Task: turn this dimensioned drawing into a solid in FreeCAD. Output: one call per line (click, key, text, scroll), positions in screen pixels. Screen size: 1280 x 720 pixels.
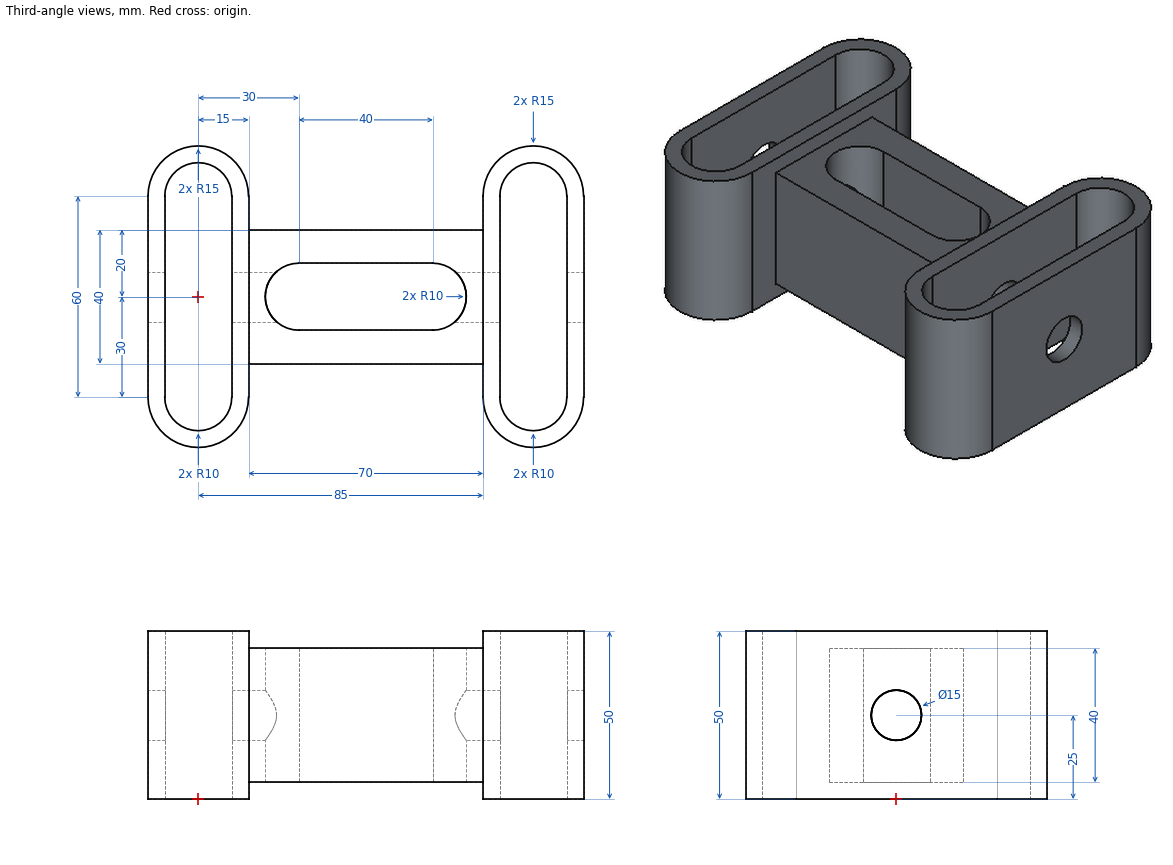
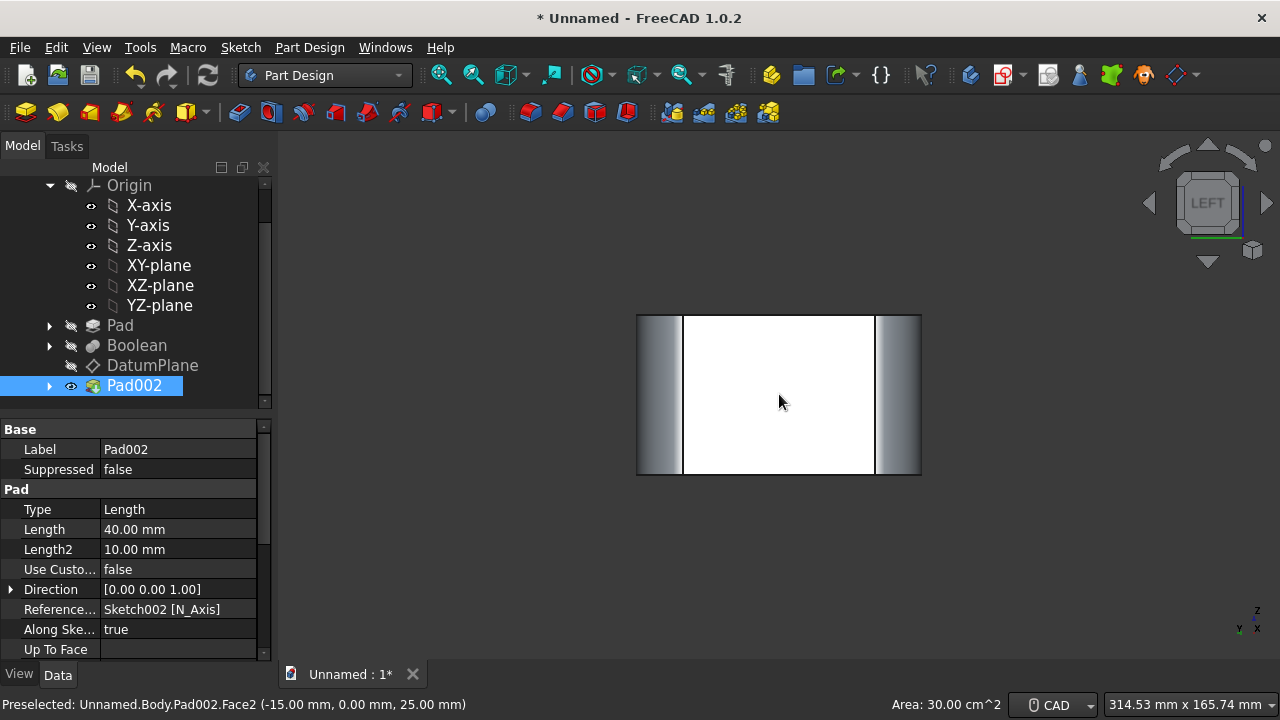
click(1004, 76)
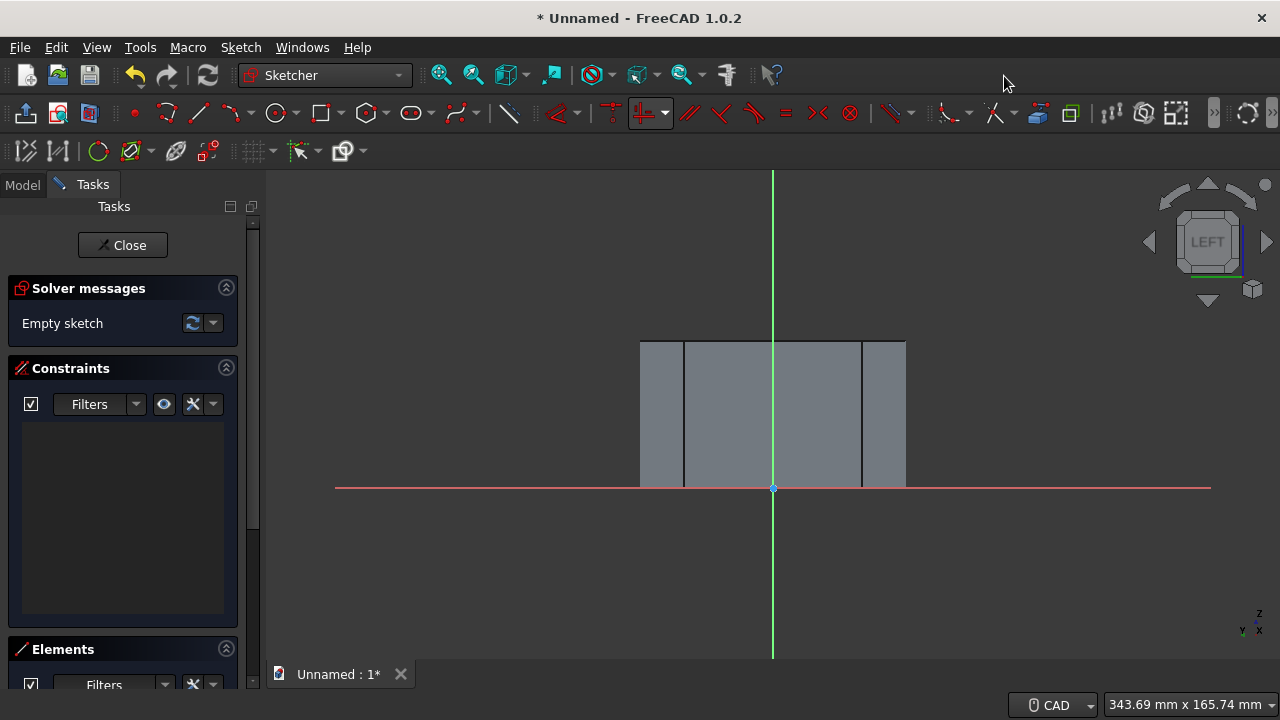
scroll(803, 451, up, 6)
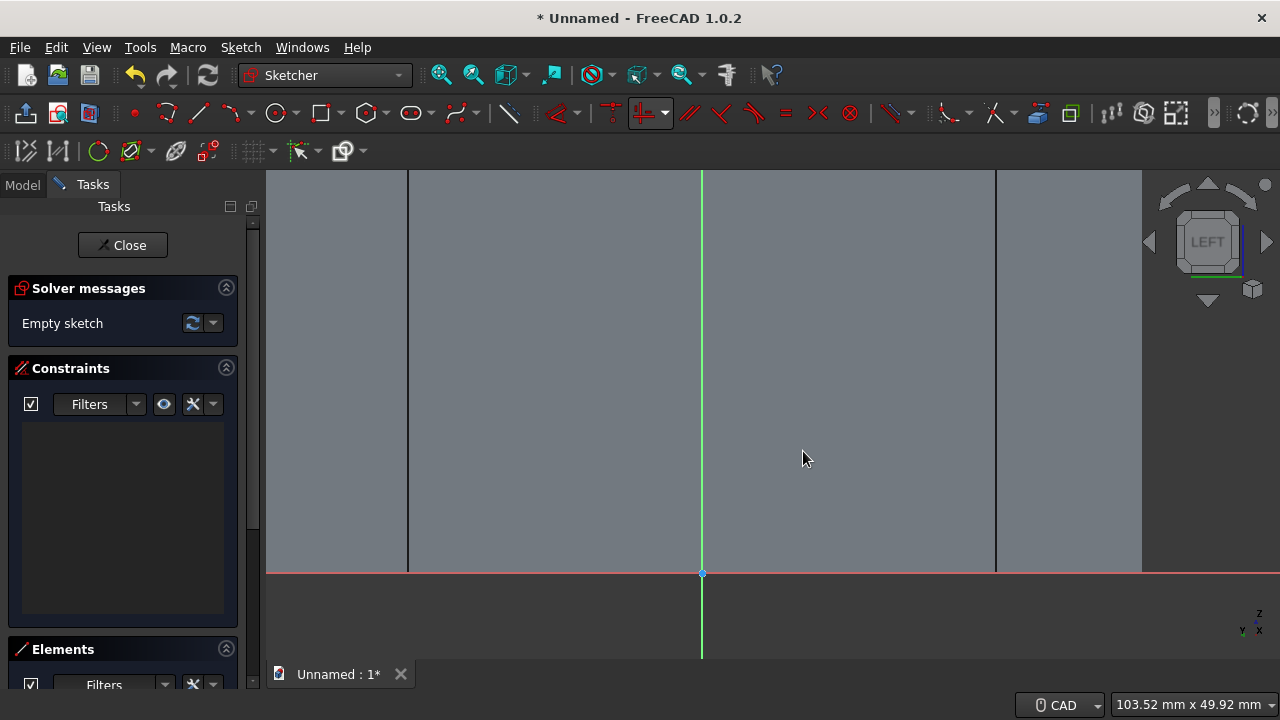
click(276, 114)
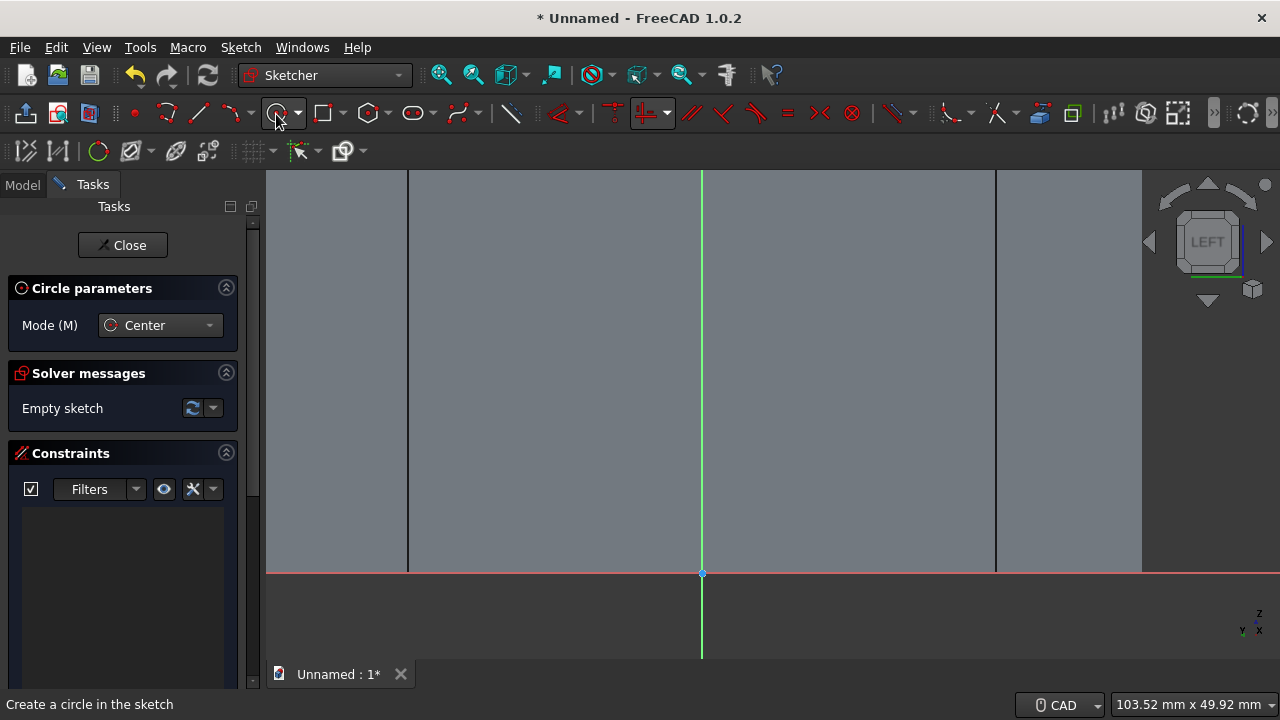
click(702, 328)
click(754, 277)
key(Escape)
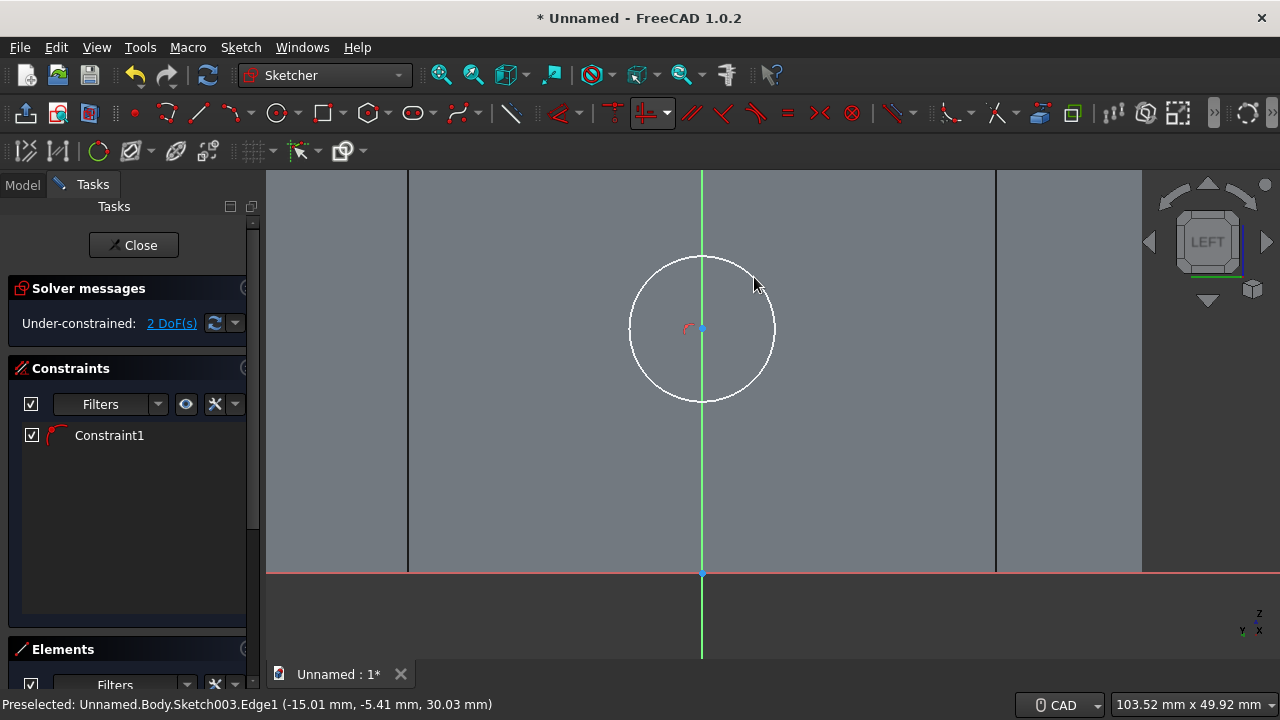
click(558, 114)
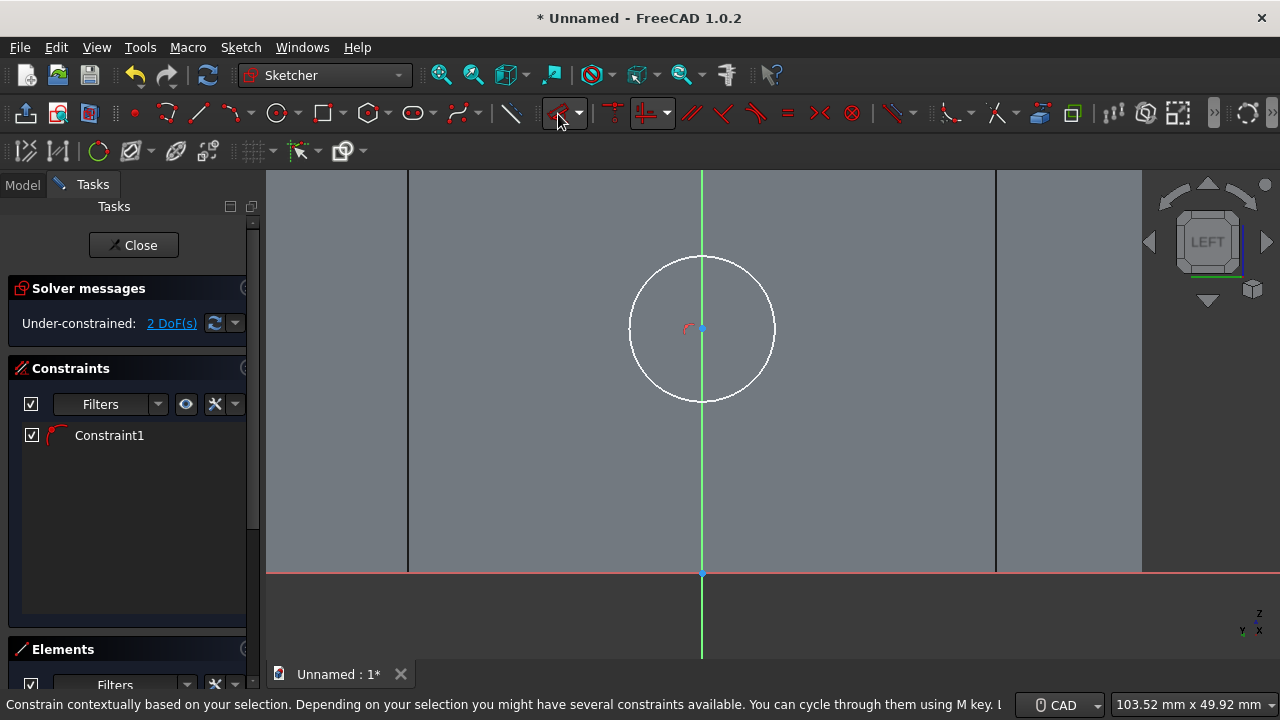
click(753, 277)
click(775, 254)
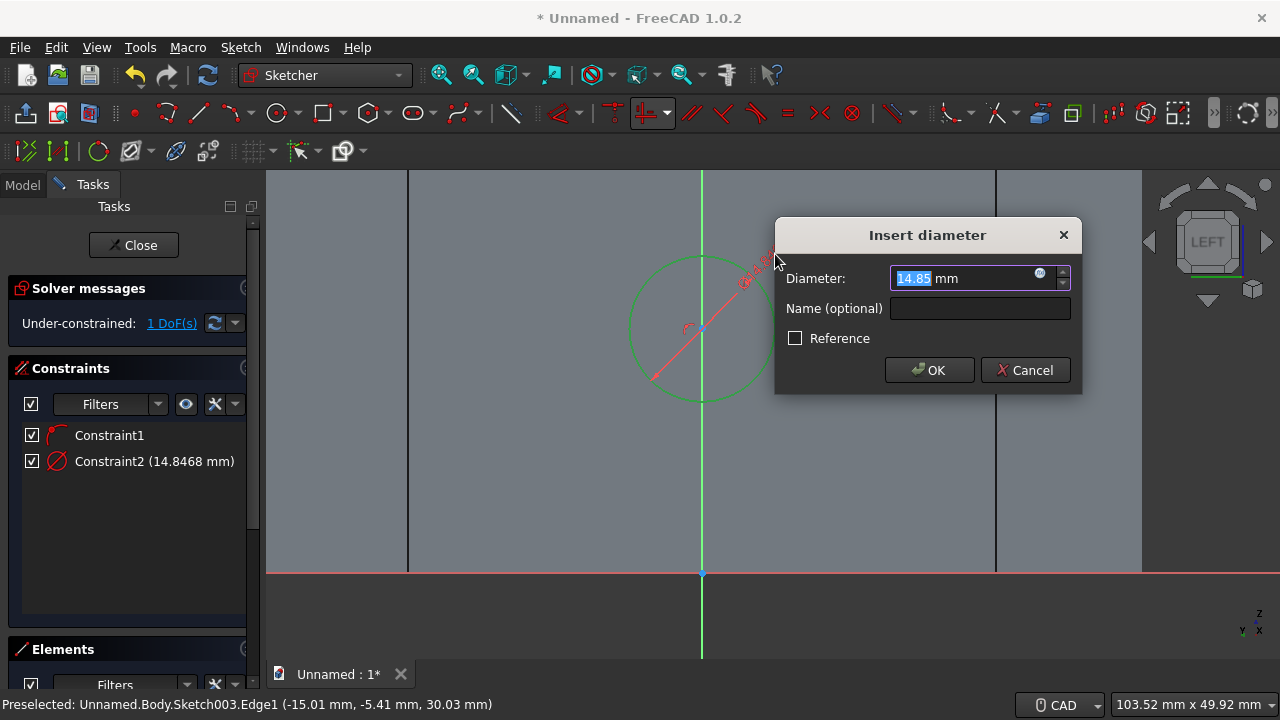
text(15)
key(Return)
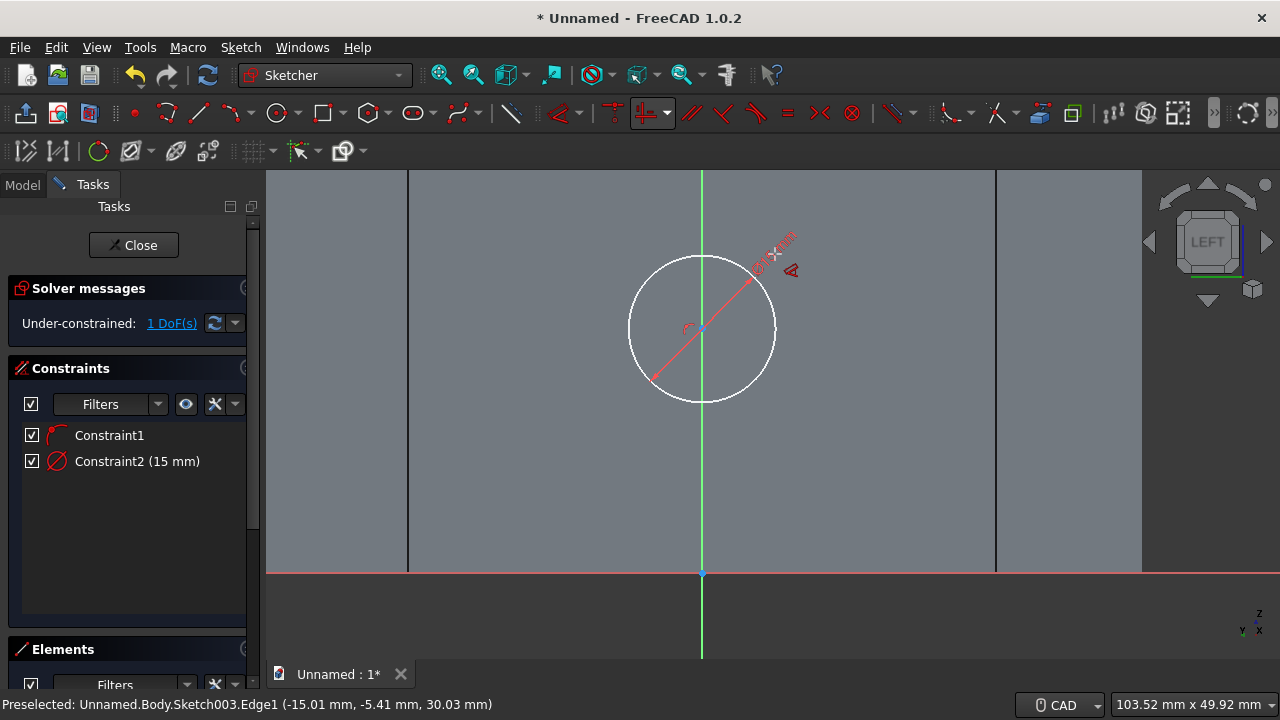
click(702, 329)
click(736, 451)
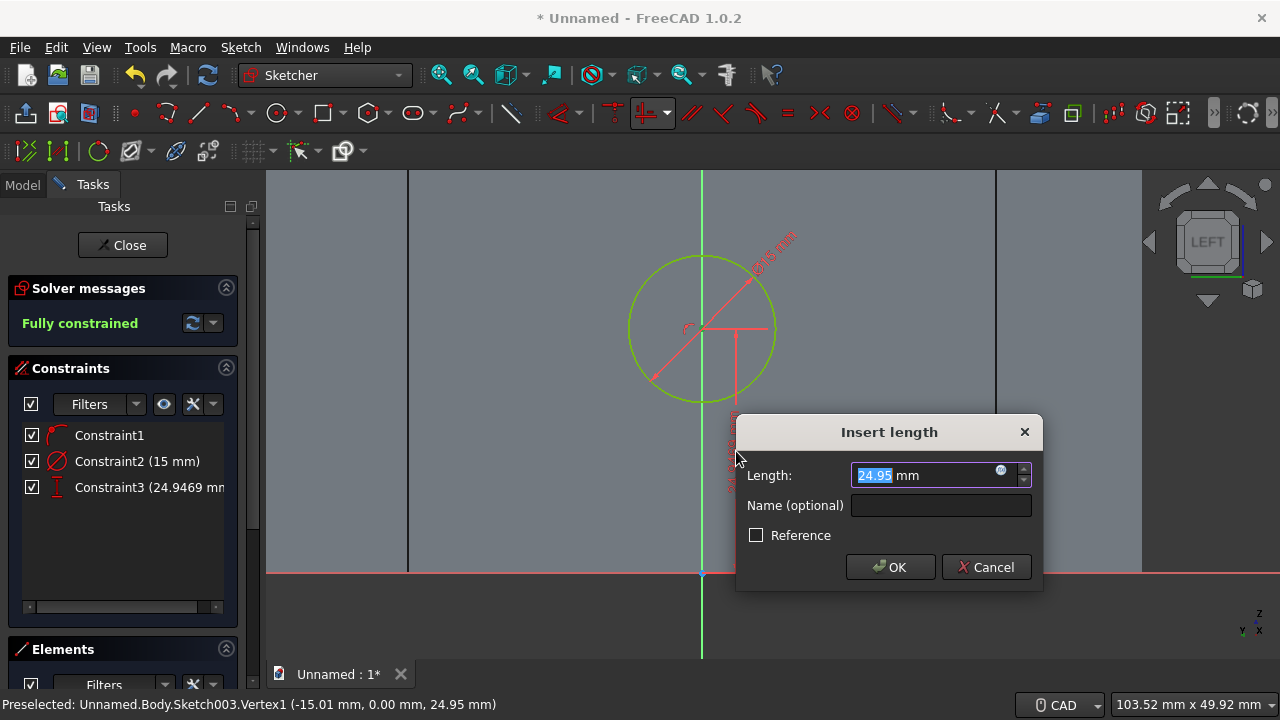
text(25)
key(Return)
key(Escape)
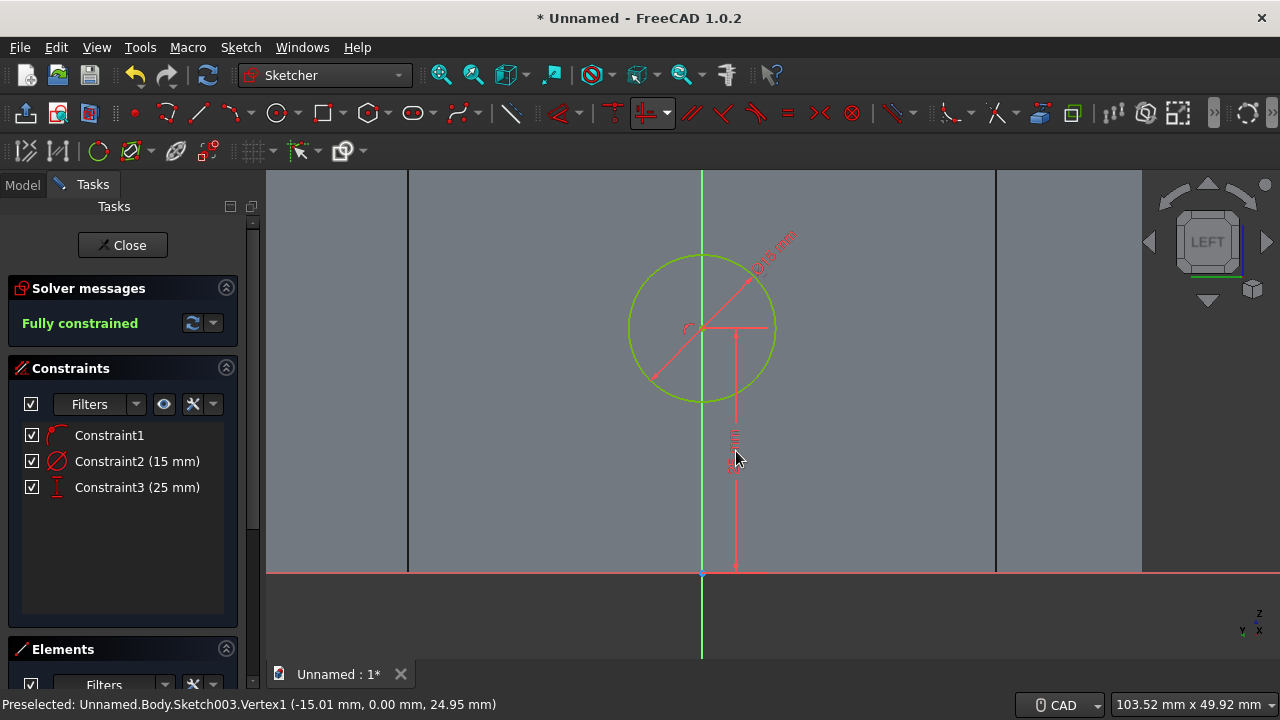
click(123, 245)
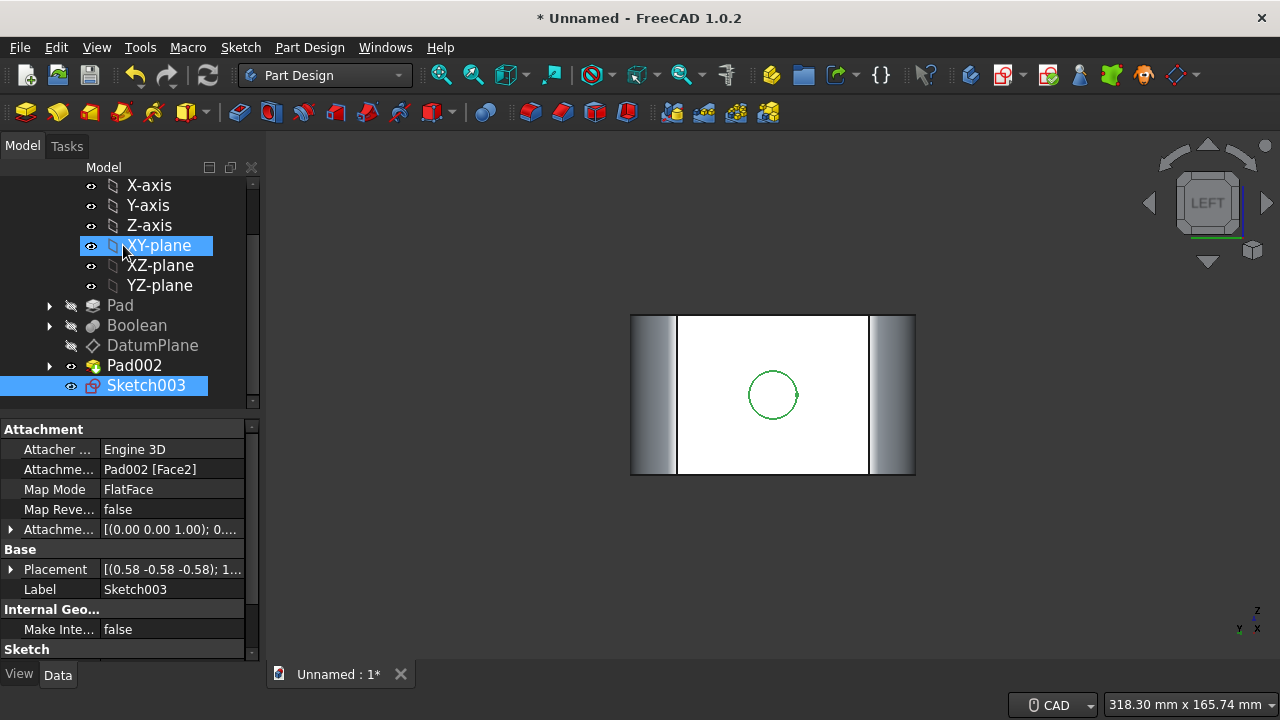
click(240, 112)